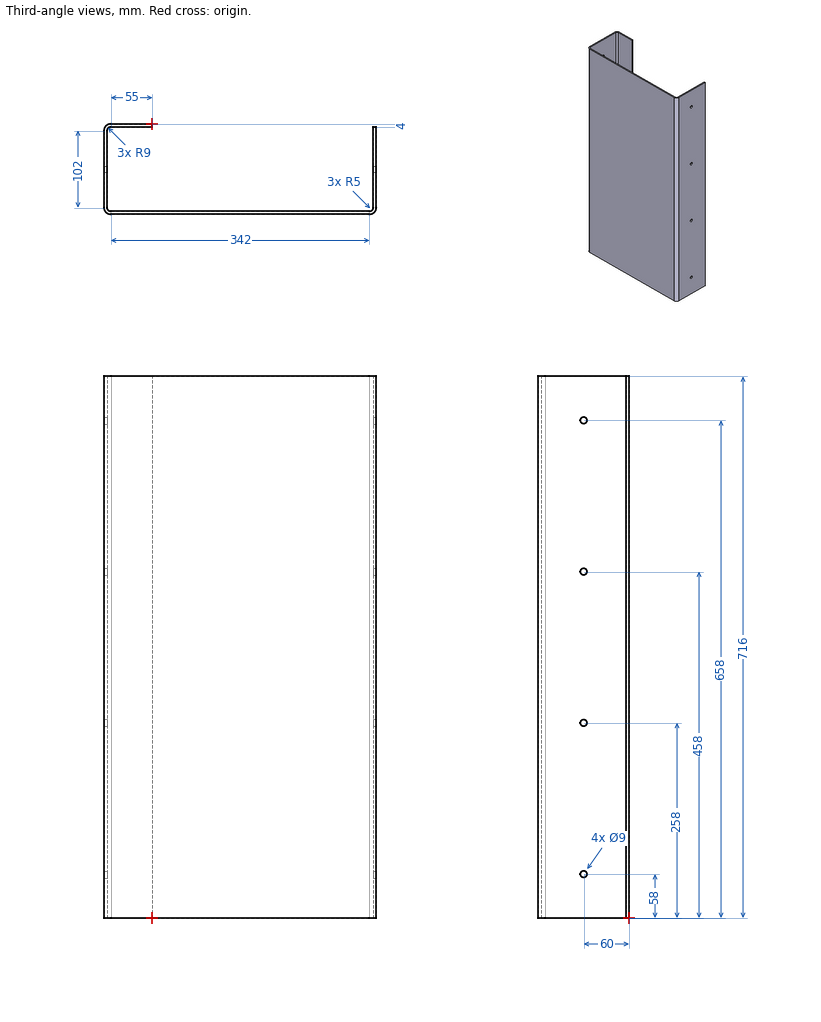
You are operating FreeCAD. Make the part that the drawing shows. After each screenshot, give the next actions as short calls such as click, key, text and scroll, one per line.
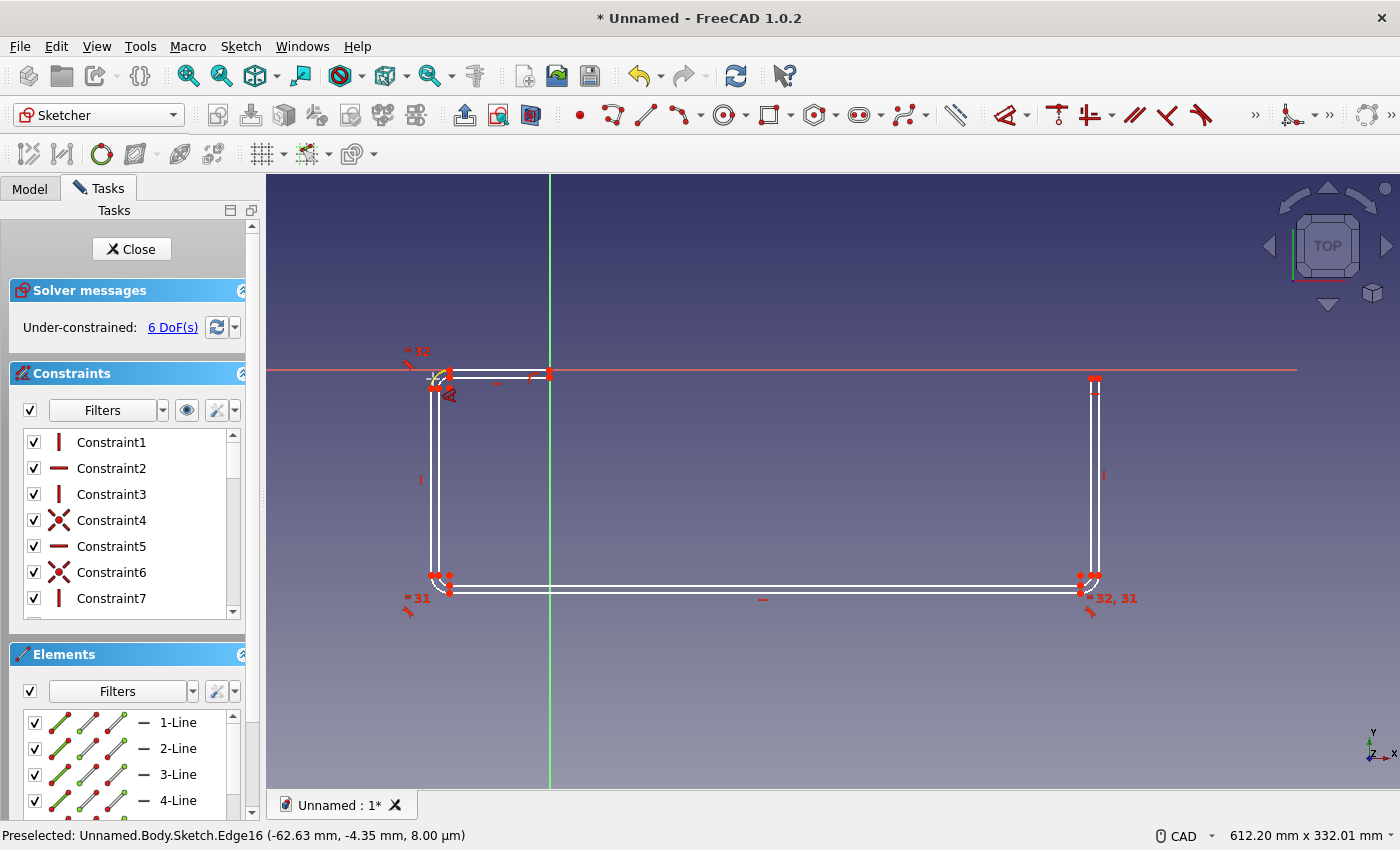
scroll(433, 583, up, 5)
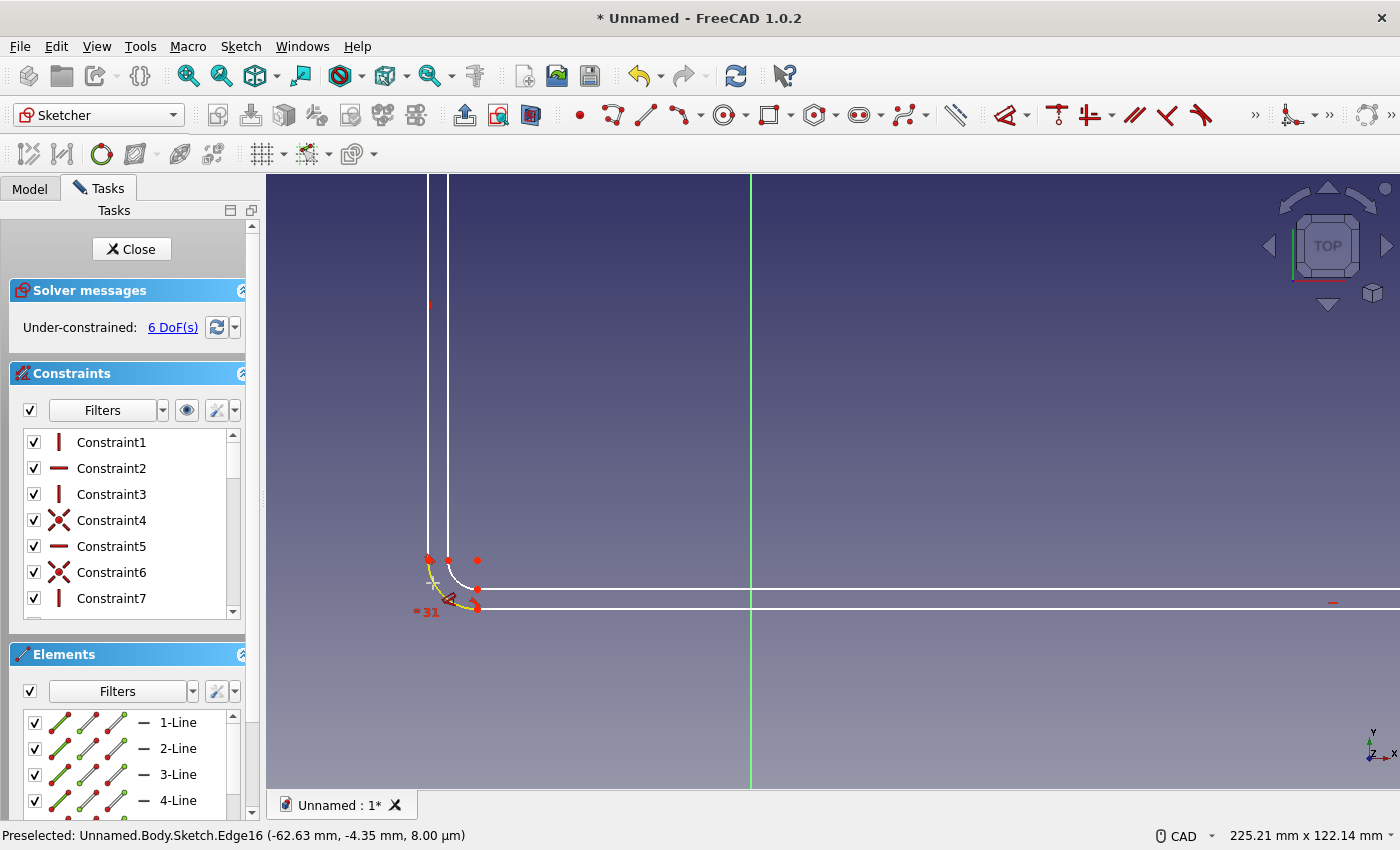
click(434, 583)
click(406, 598)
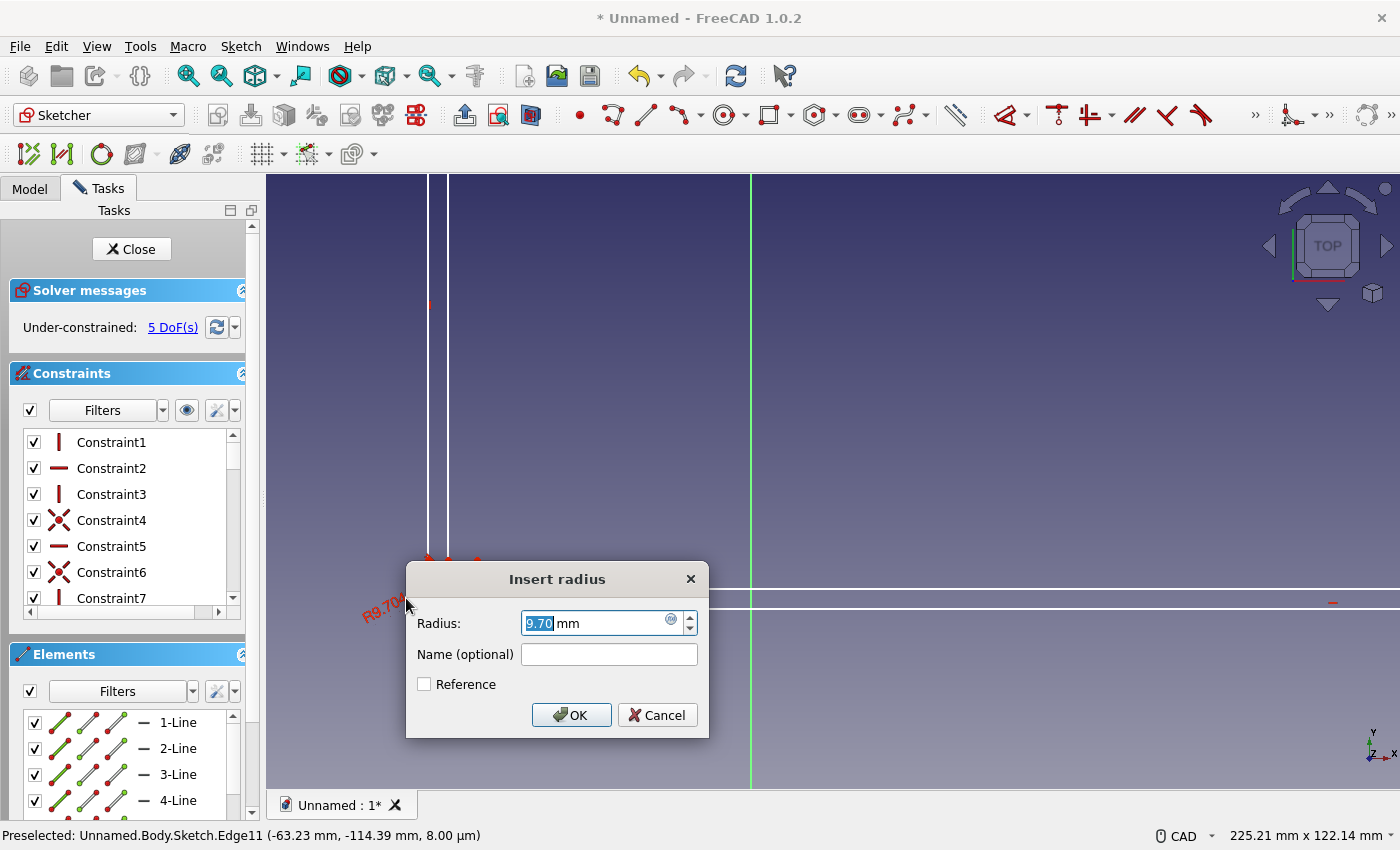
text(9)
key(Return)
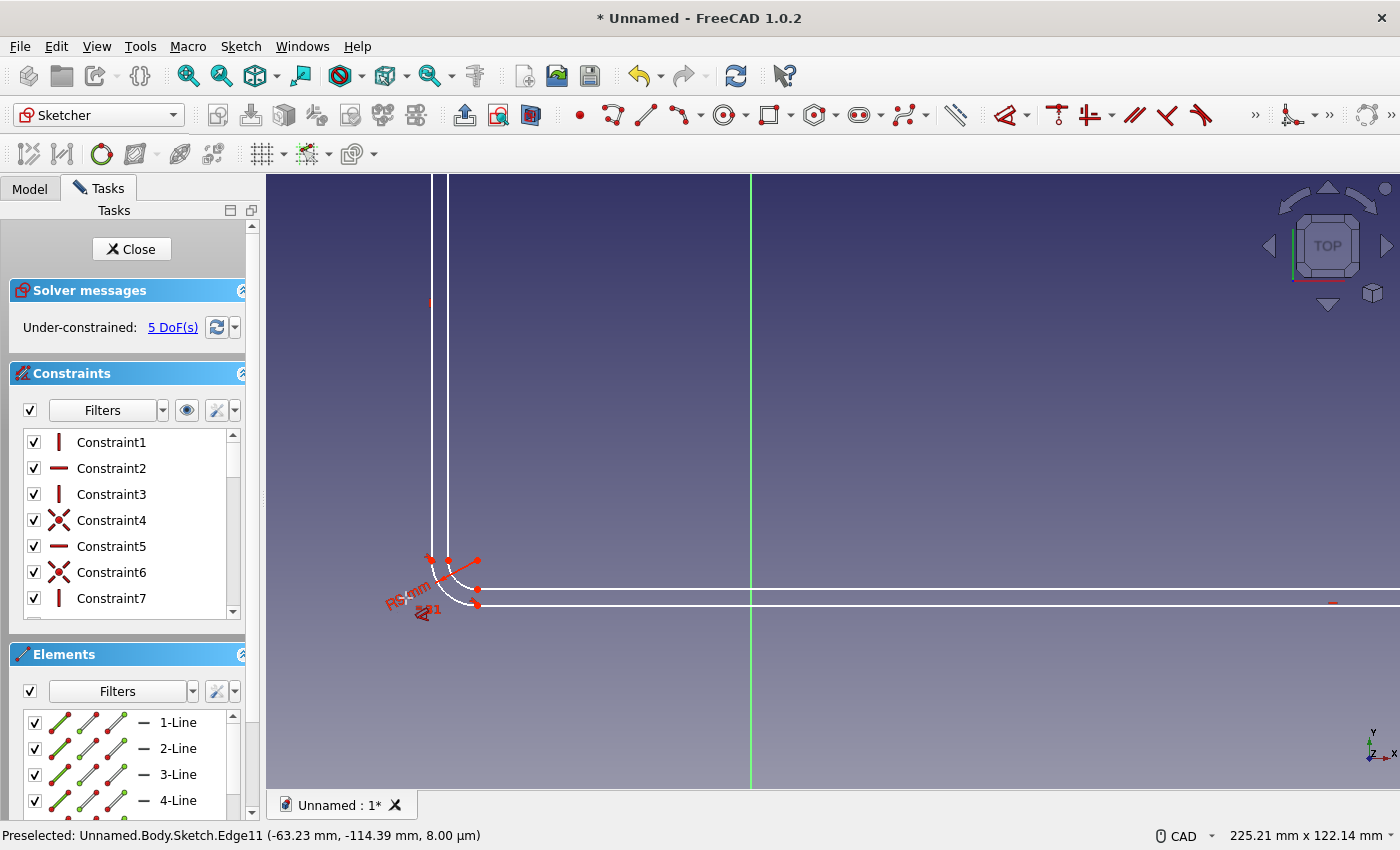
scroll(433, 584, down, 5)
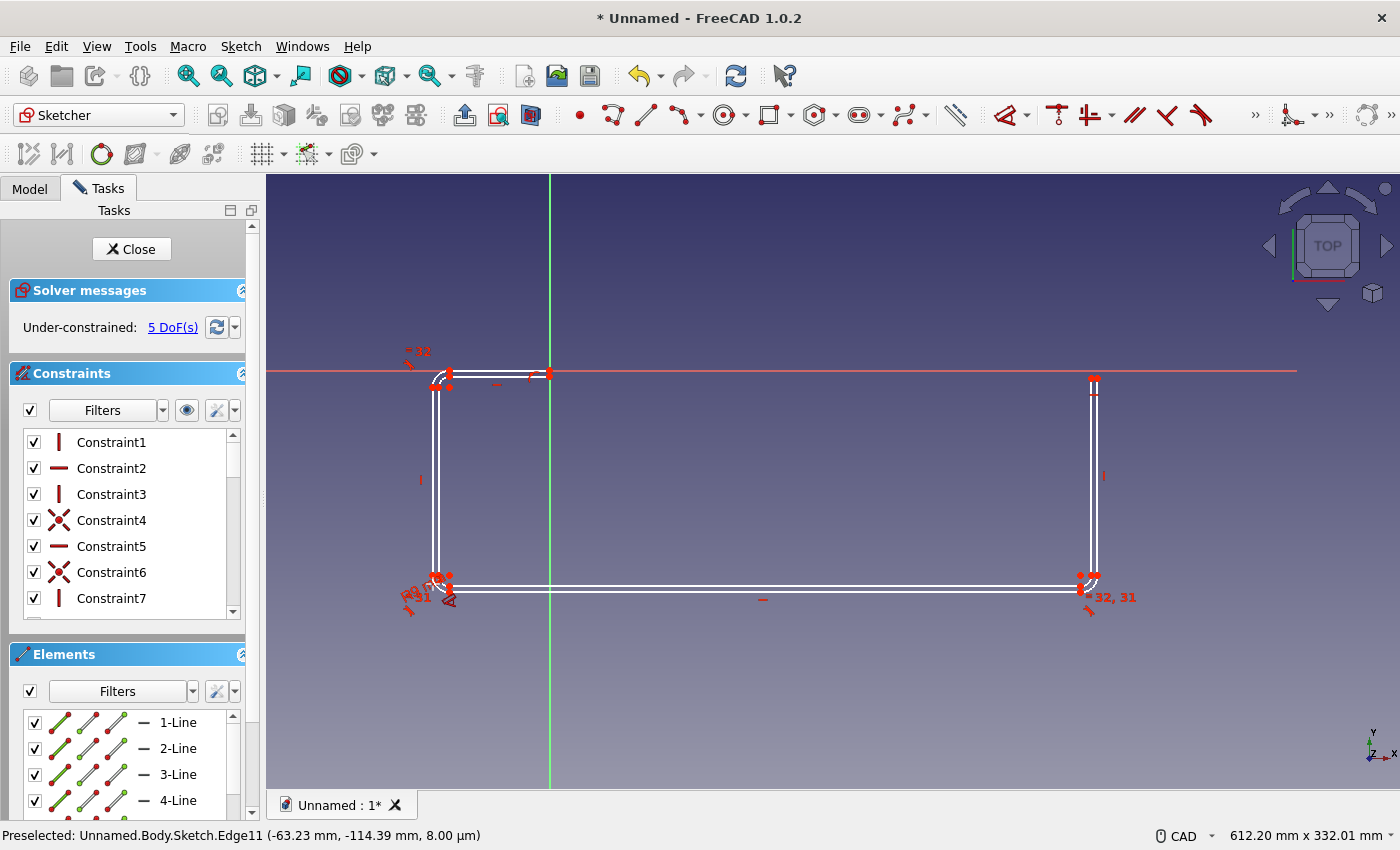
scroll(1086, 585, up, 8)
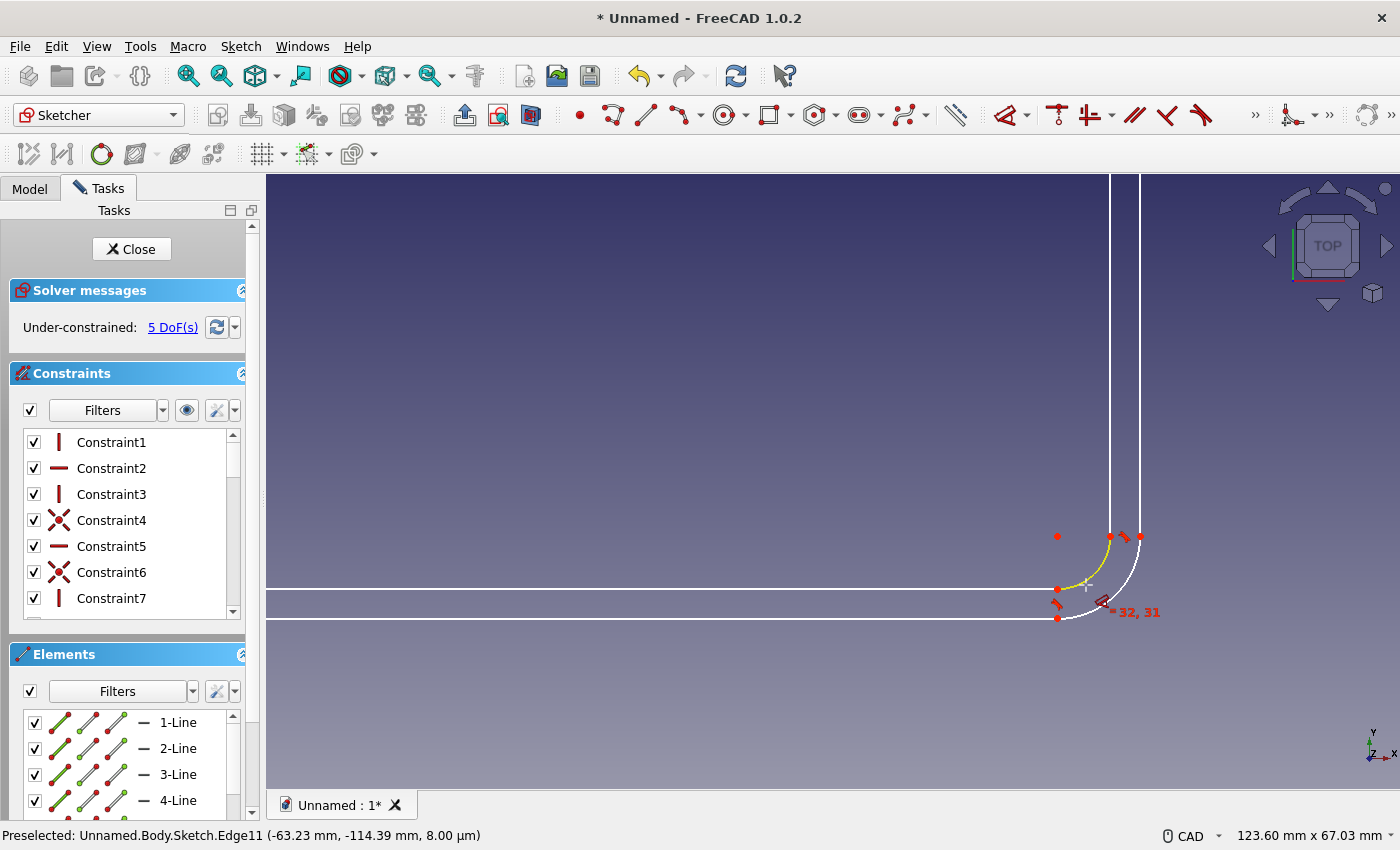
click(1081, 583)
click(982, 574)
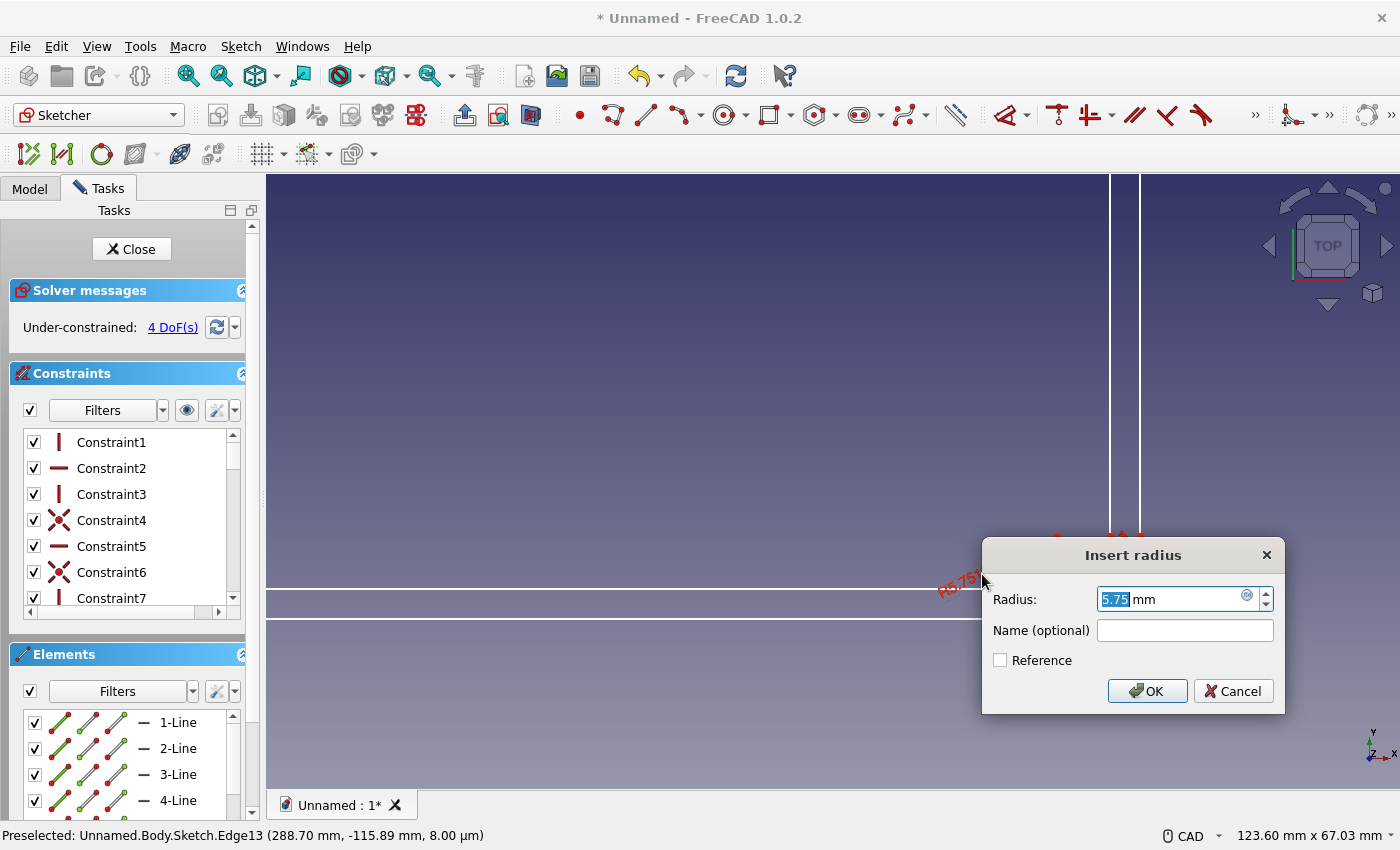
text(5)
key(Return)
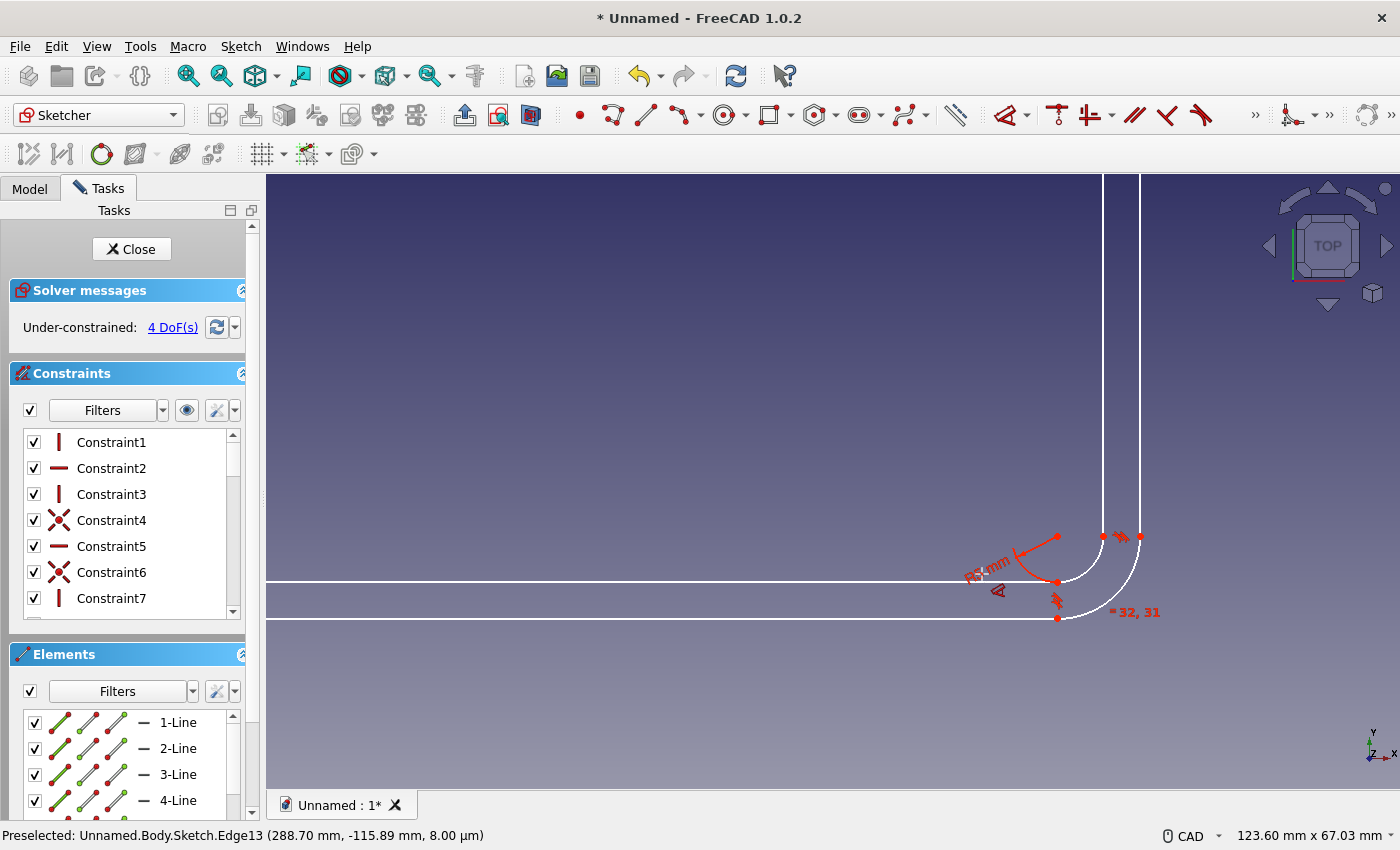
scroll(1086, 585, down, 8)